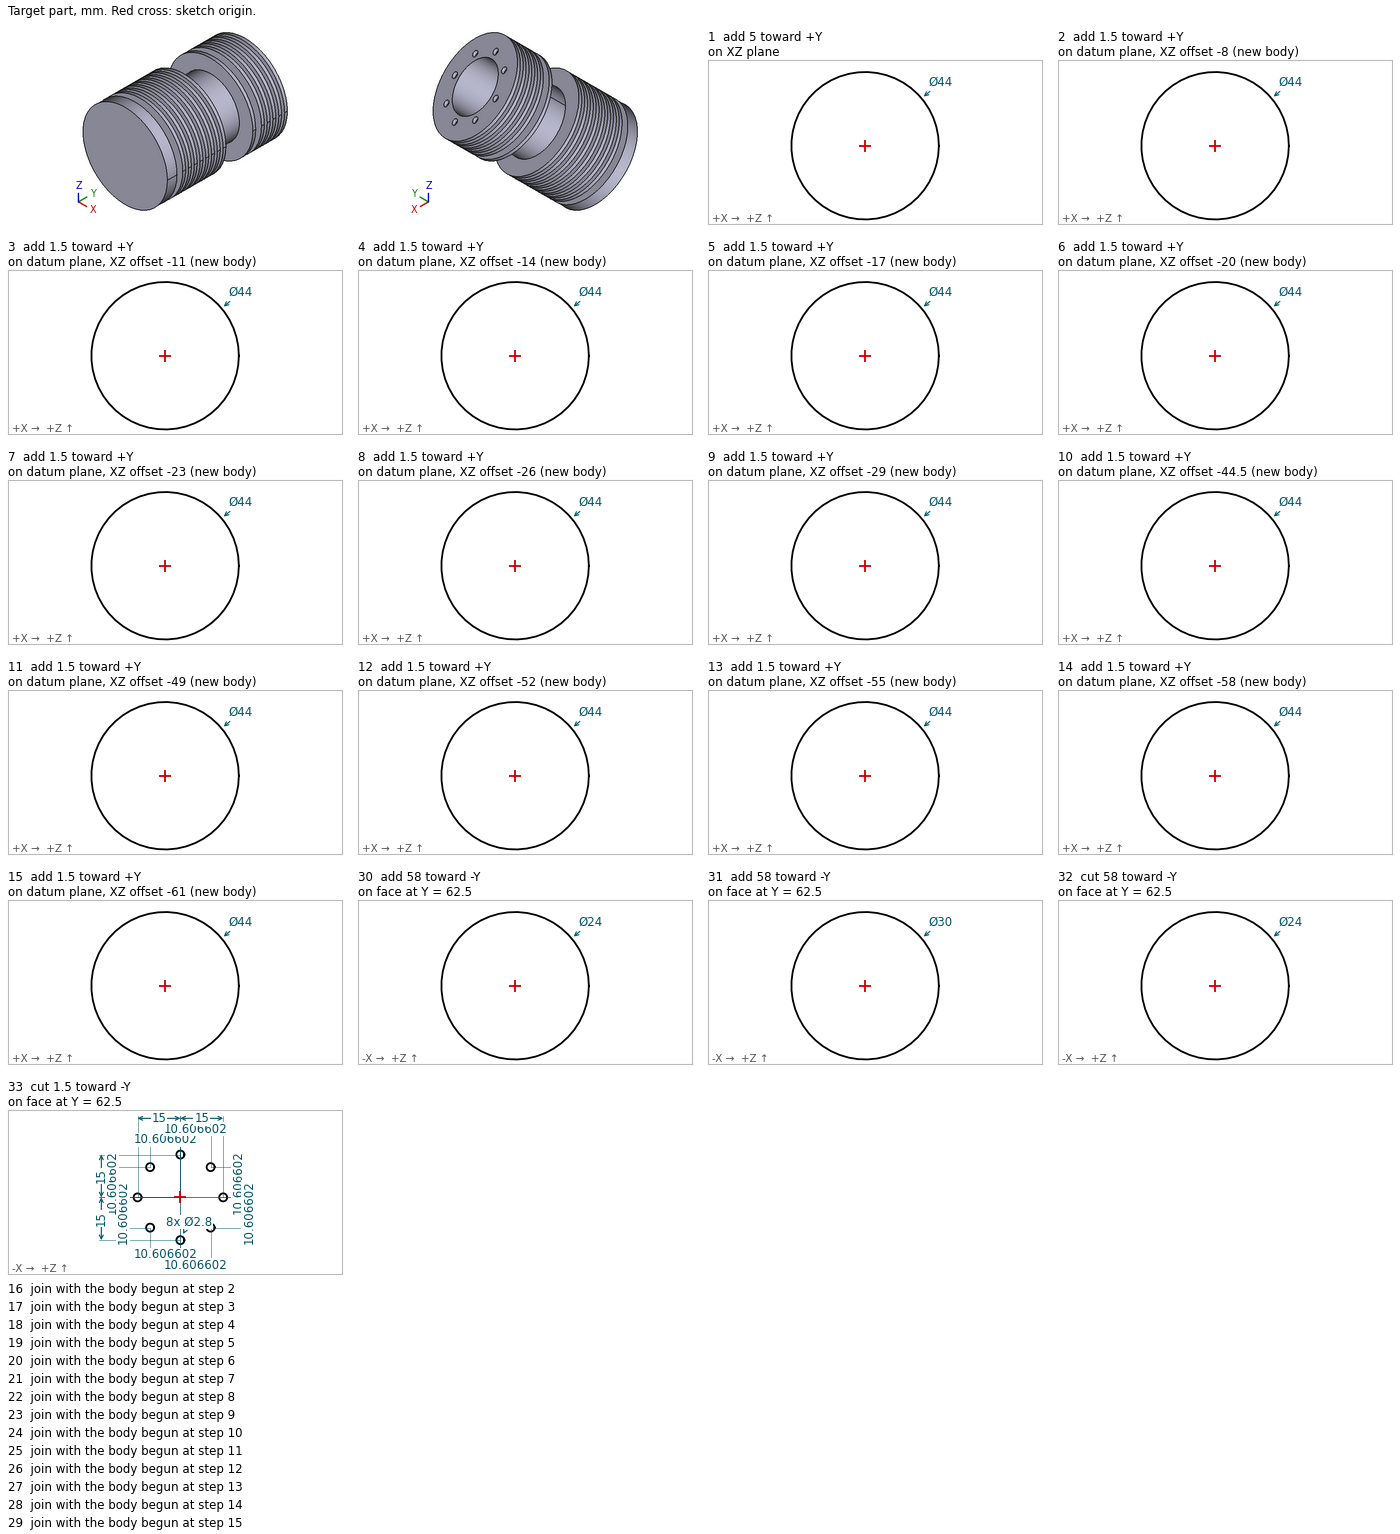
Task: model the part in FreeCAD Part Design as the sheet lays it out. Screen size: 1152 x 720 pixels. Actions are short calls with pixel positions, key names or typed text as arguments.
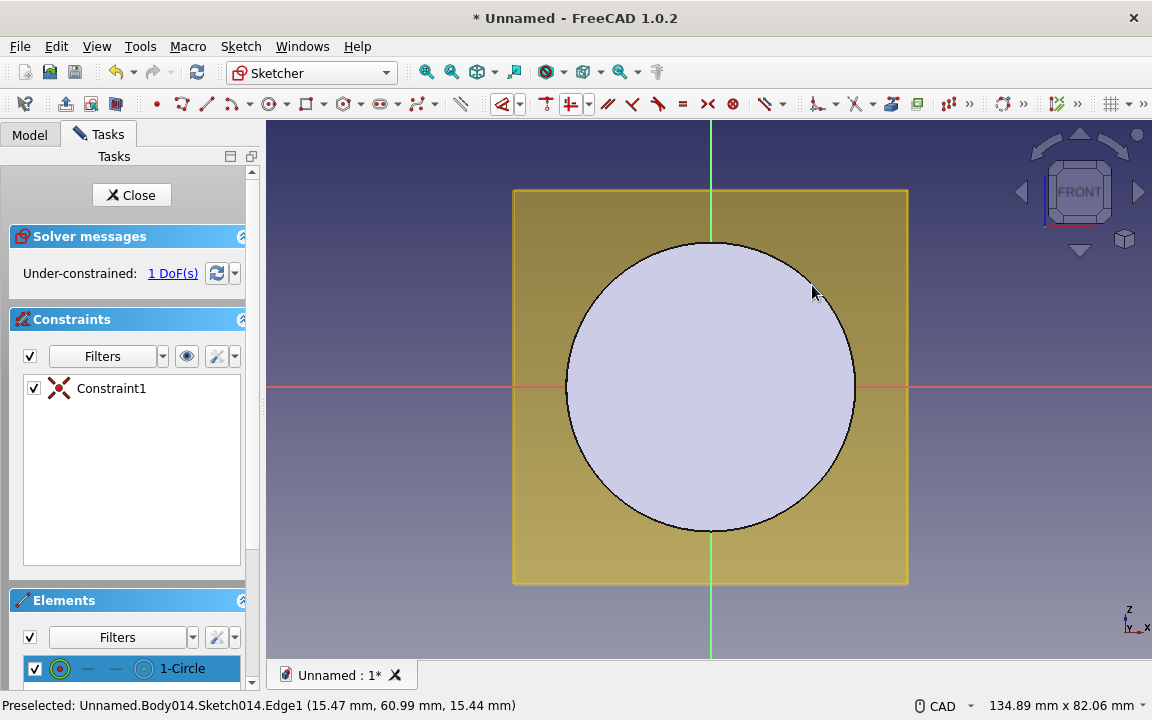
key(k)
key(o)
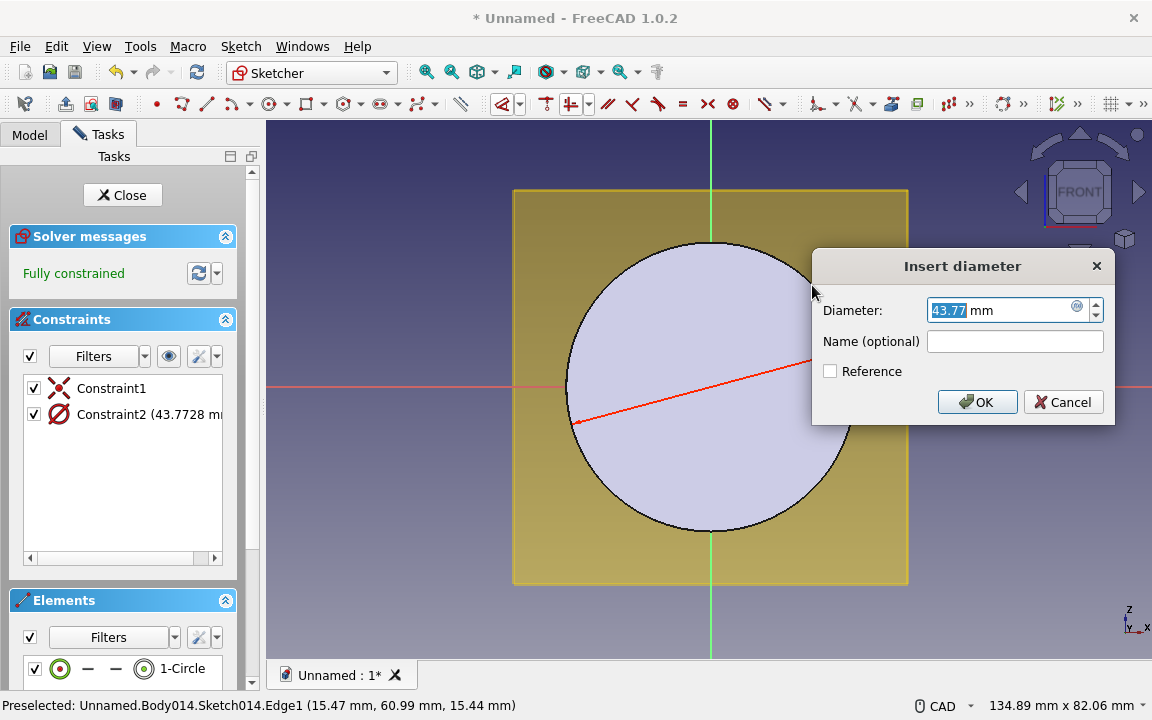
text(44)
key(Return)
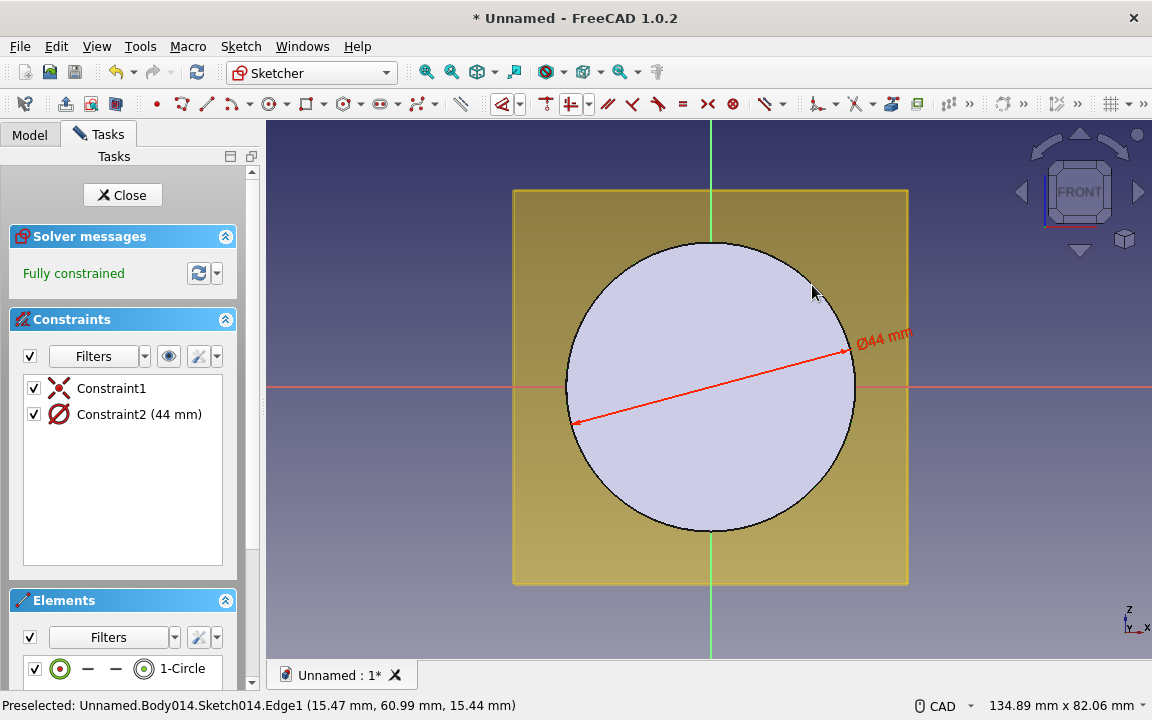
click(123, 195)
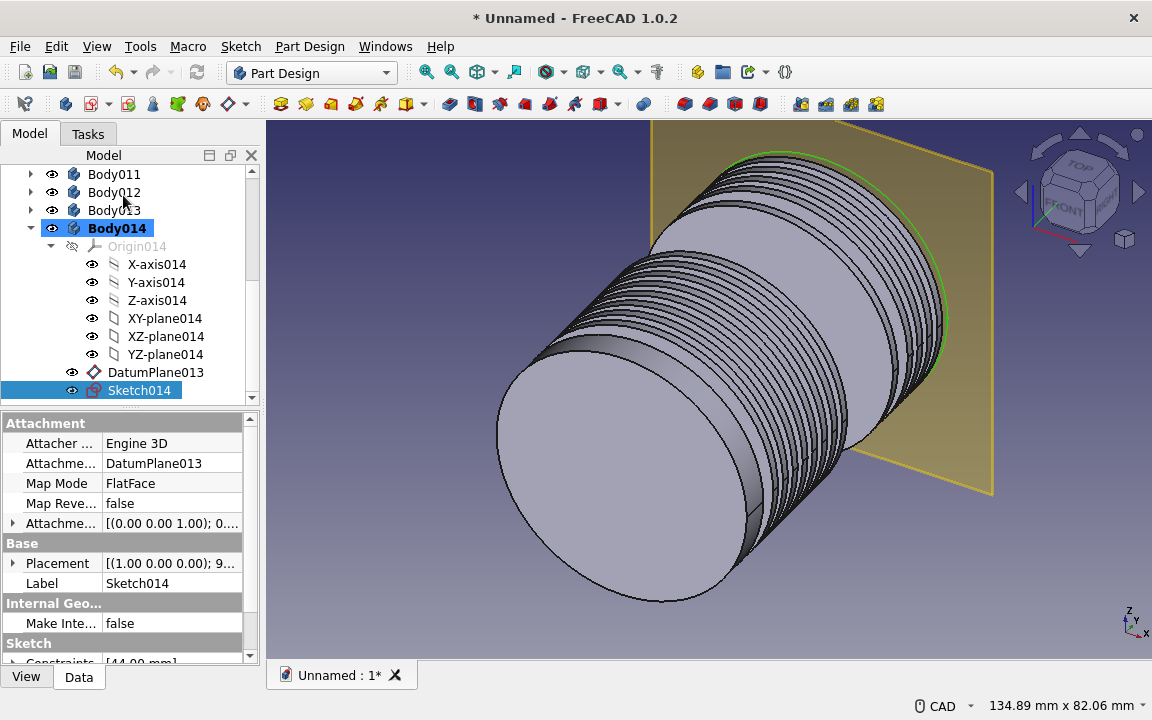
click(281, 104)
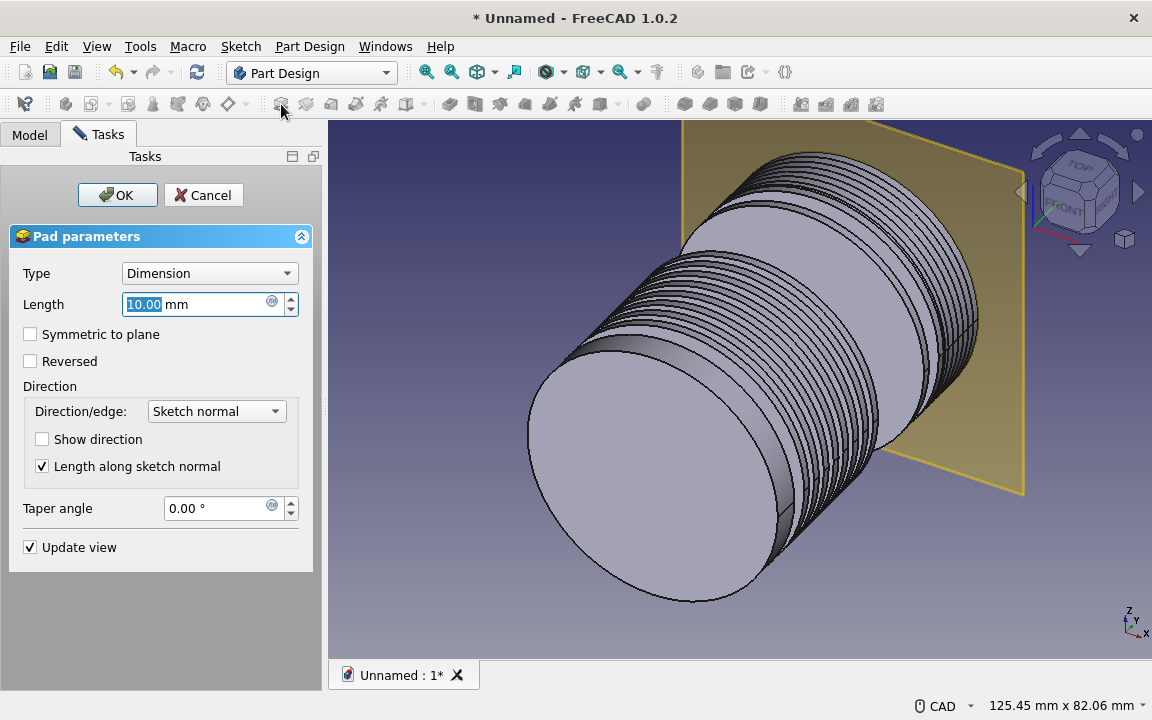
text(1.5)
key(Tab)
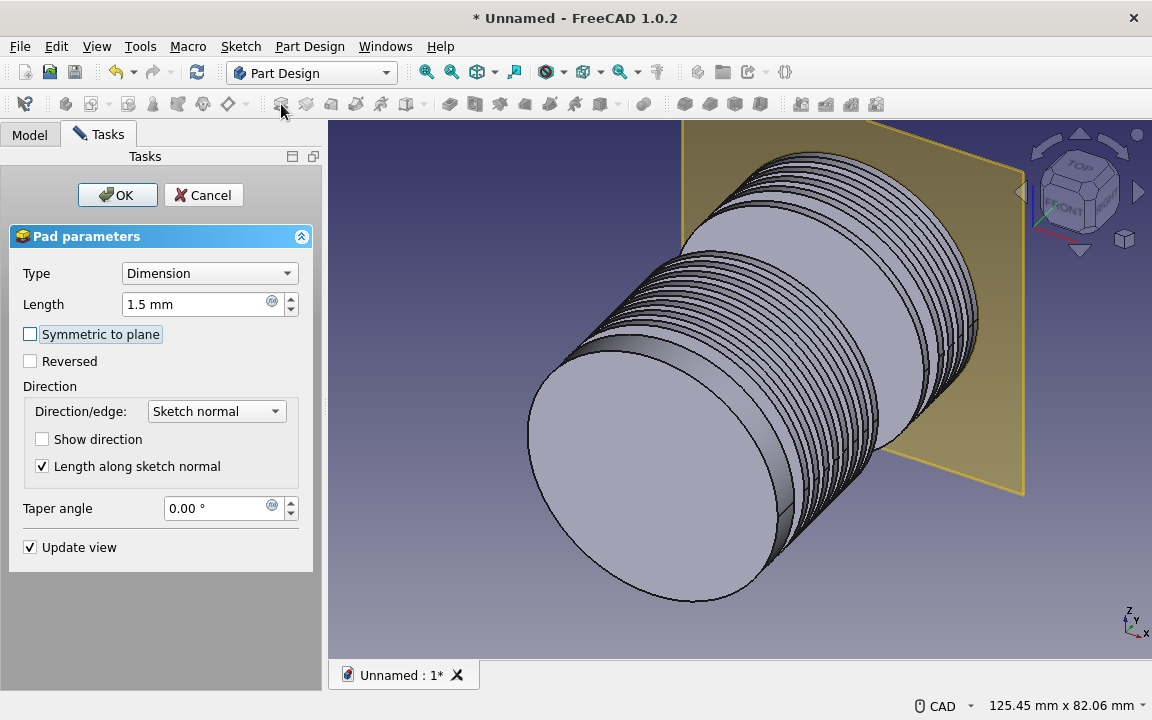
click(31, 361)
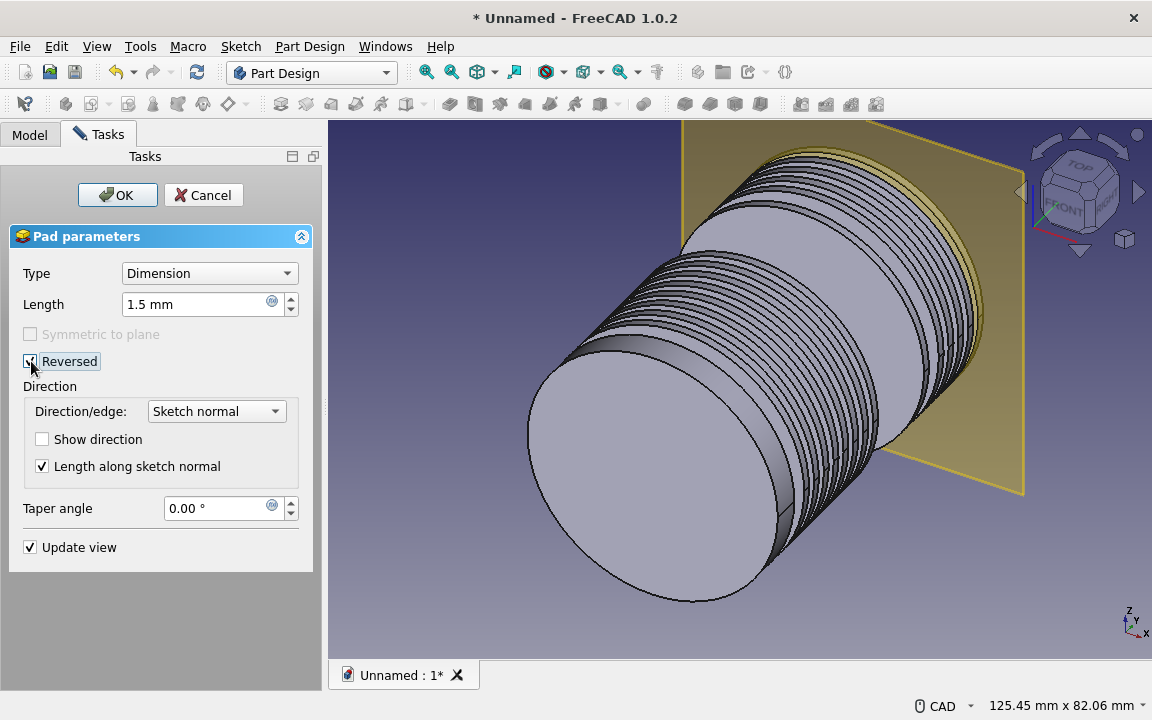
click(118, 195)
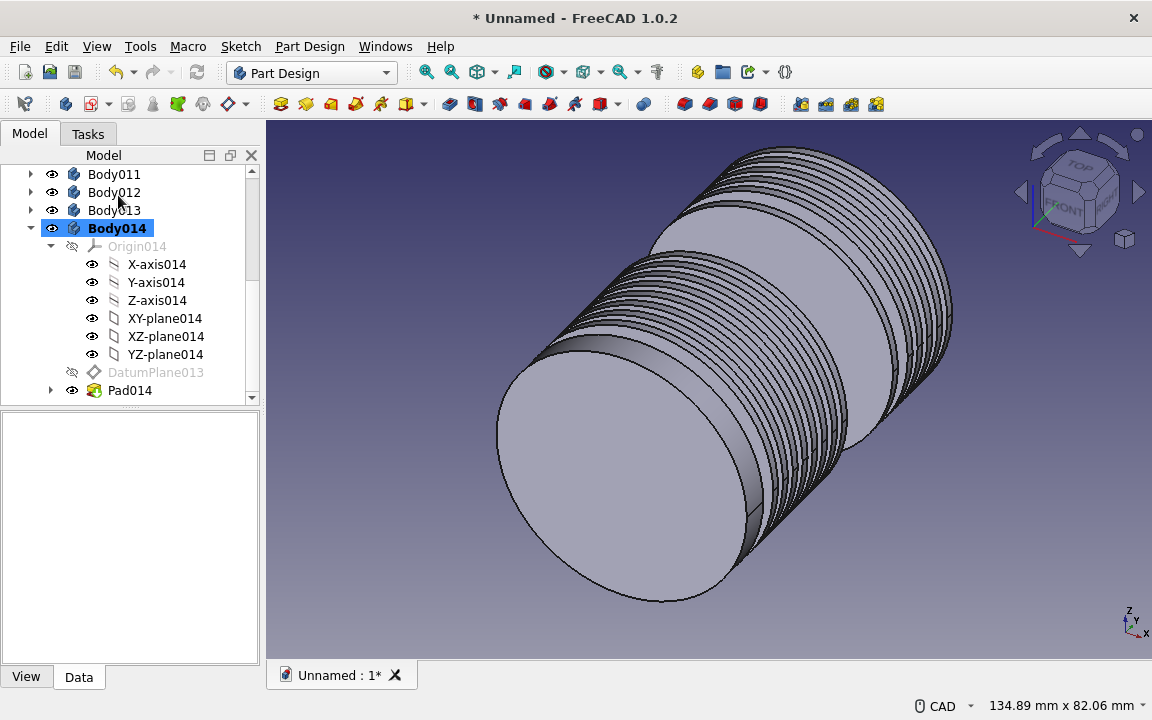
key(v)
key(f)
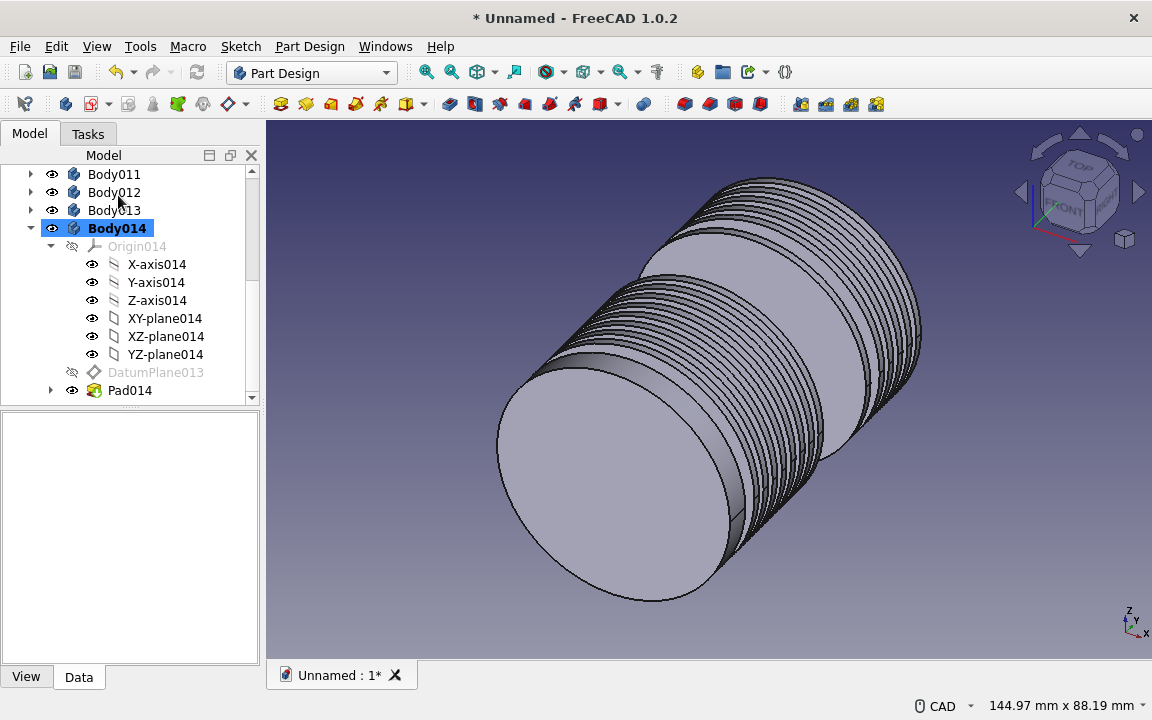
scroll(121, 278, down, 3)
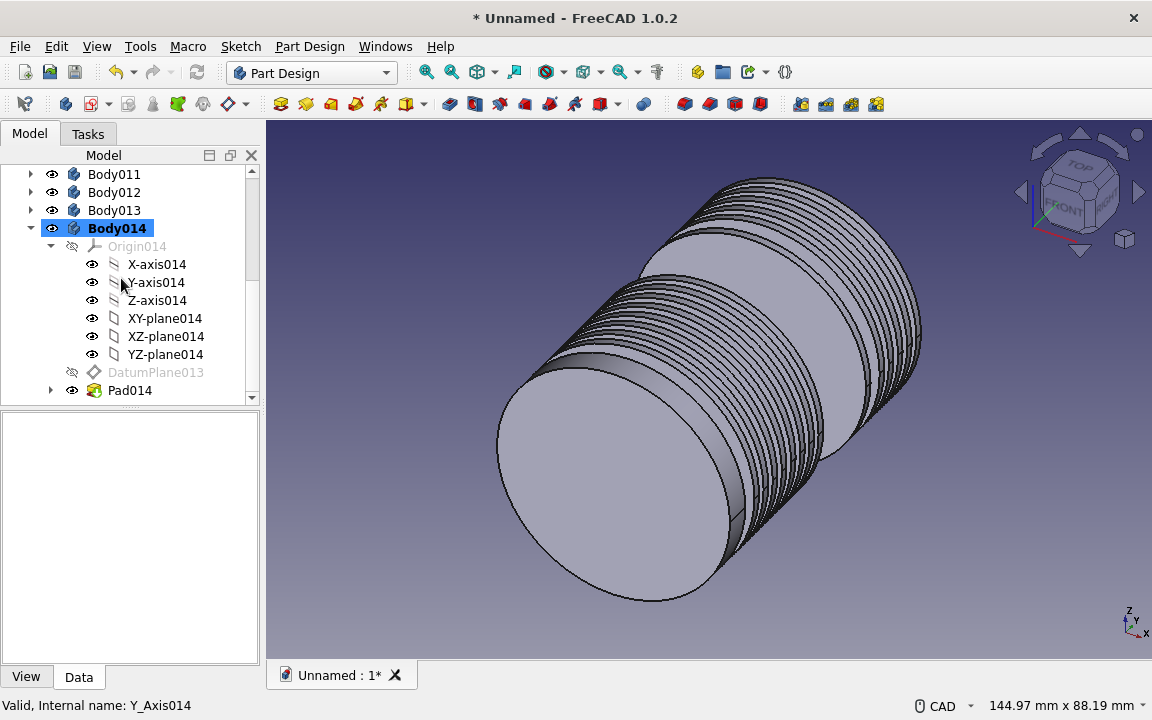
scroll(121, 278, up, 15)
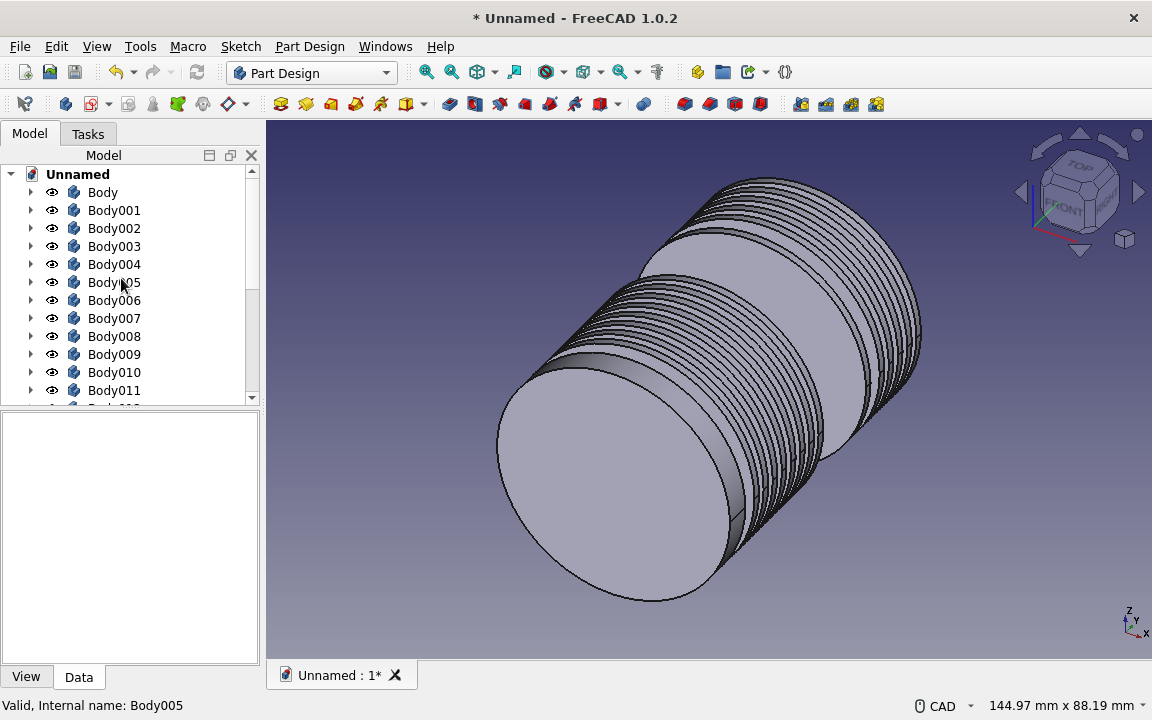
double_click(97, 192)